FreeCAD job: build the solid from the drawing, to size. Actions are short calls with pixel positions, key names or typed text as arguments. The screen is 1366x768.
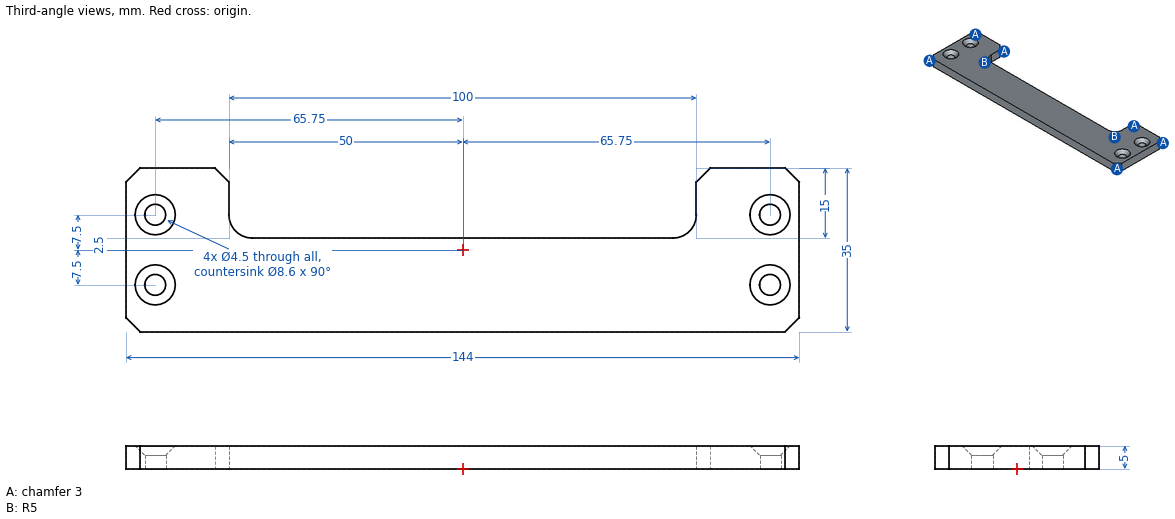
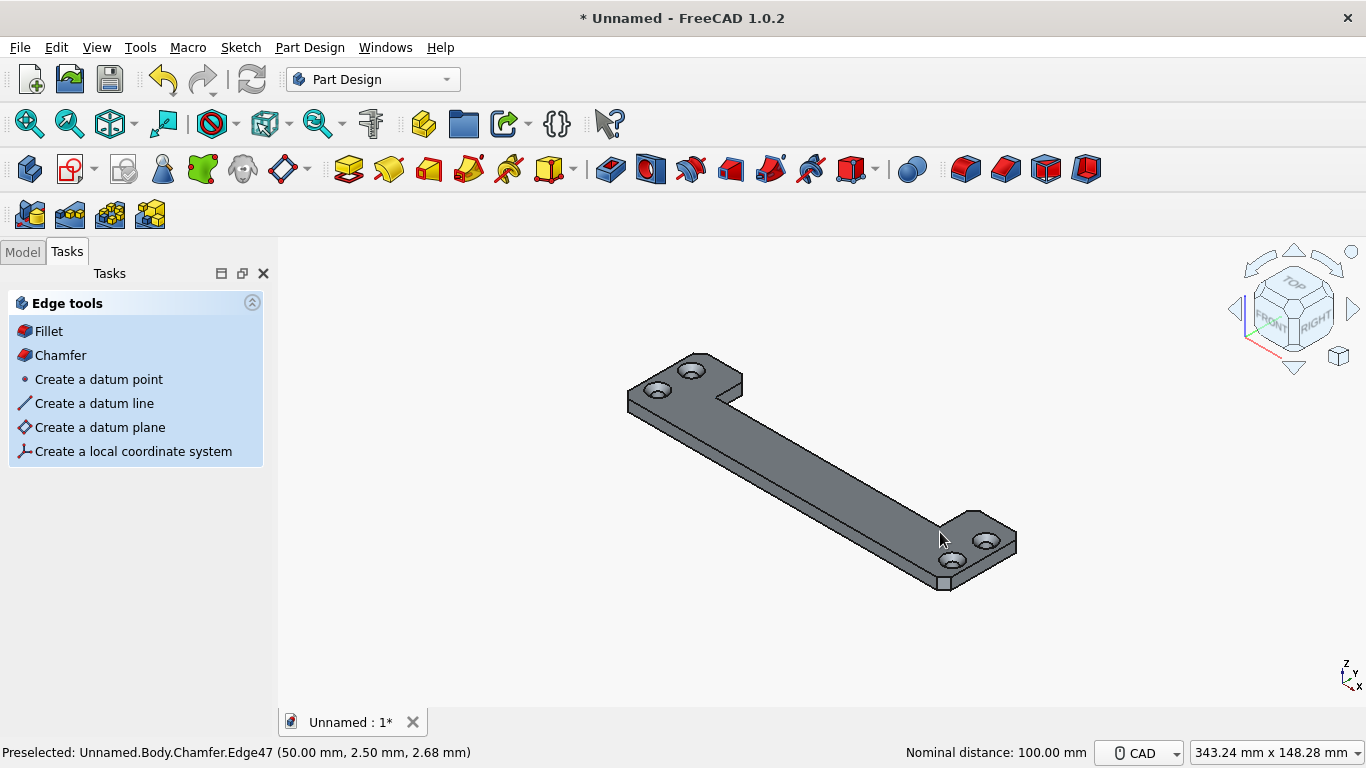
click(966, 170)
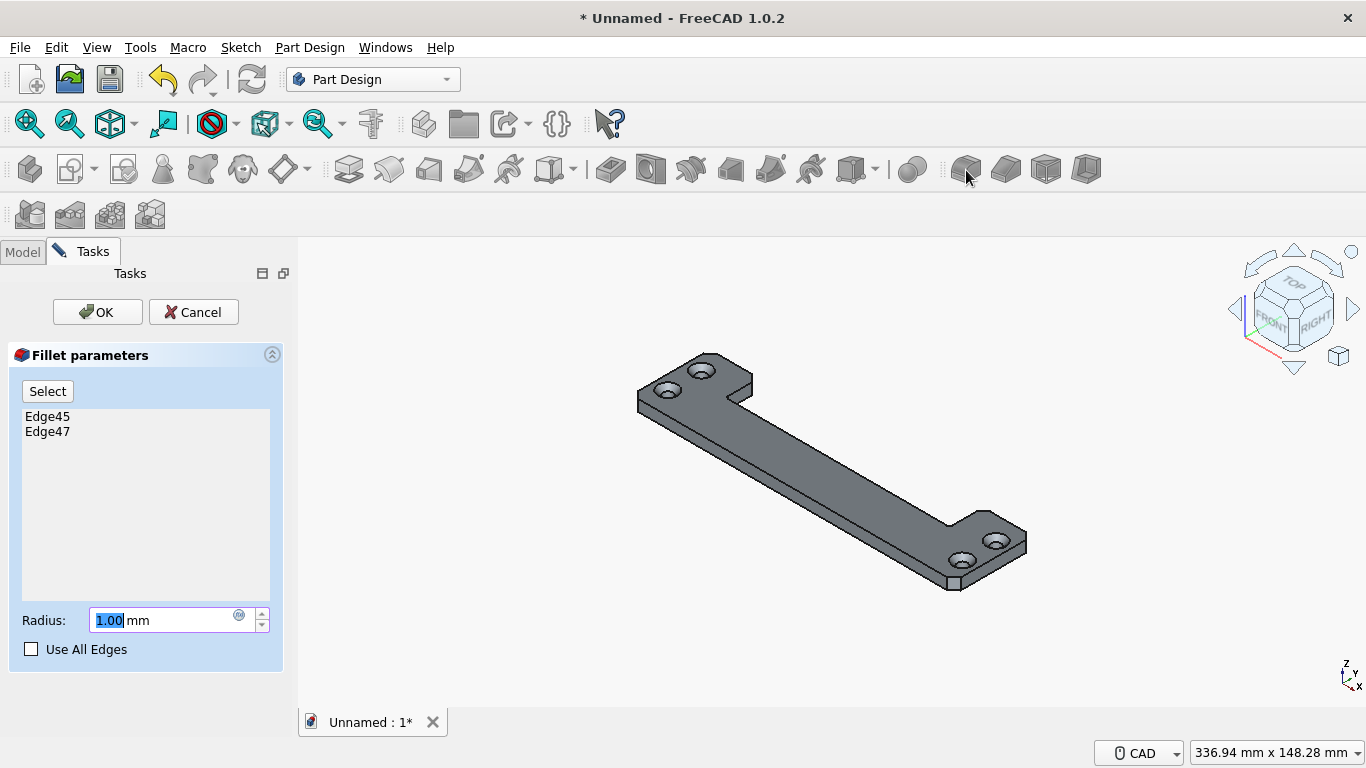
text(5)
key(Tab)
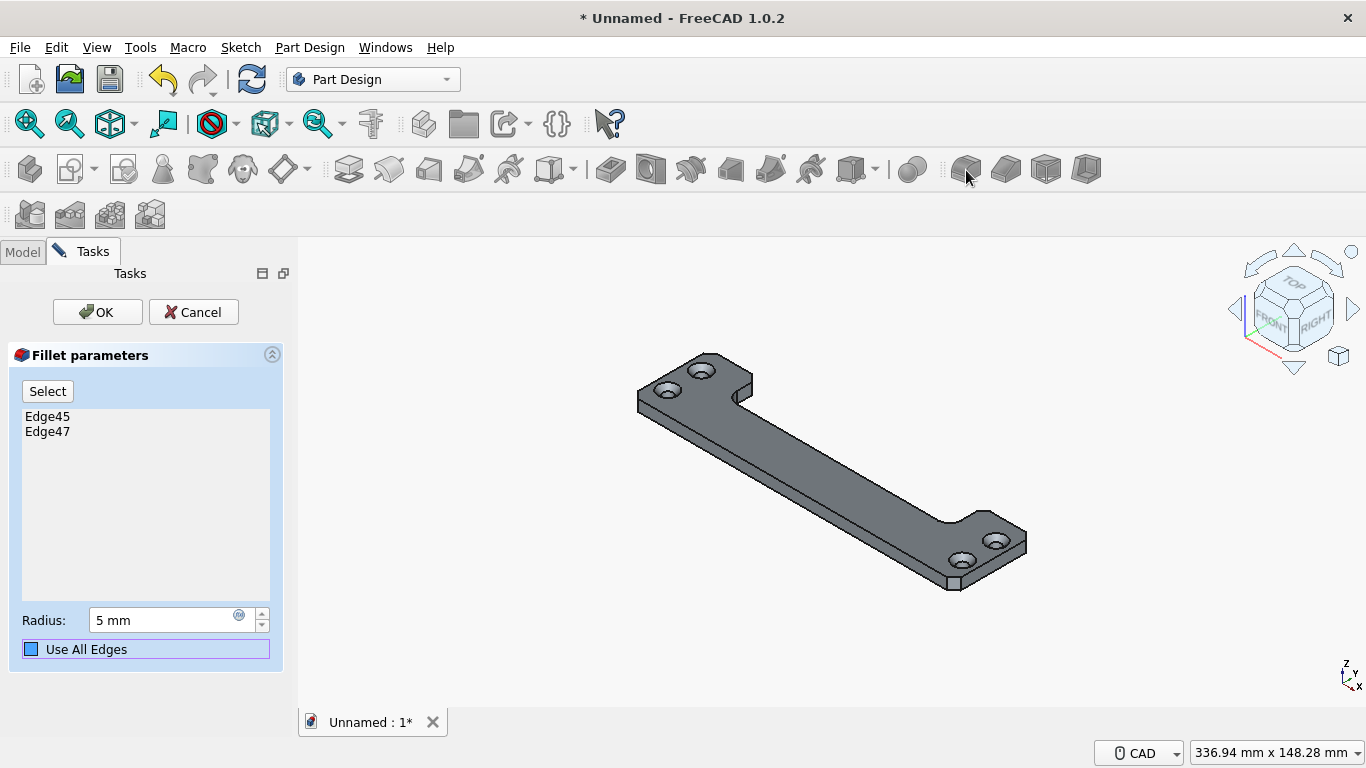
click(98, 312)